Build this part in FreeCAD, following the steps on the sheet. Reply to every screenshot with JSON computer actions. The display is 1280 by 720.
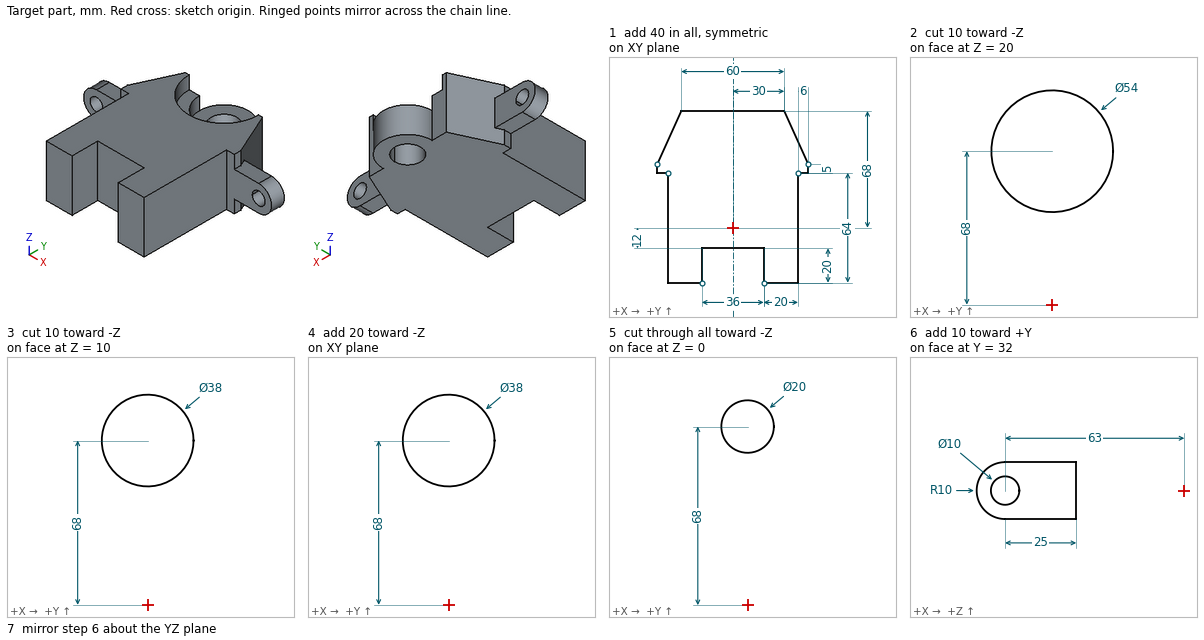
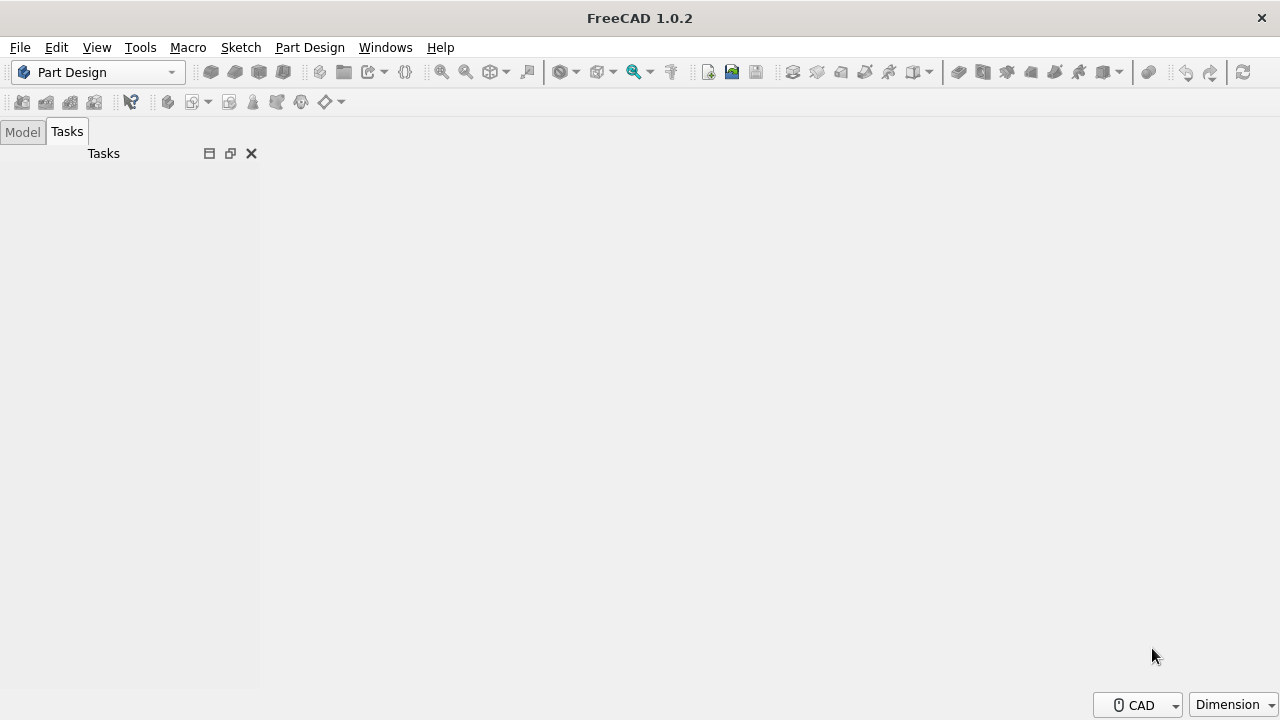
{"action": "left_click", "coordinate": [708, 72]}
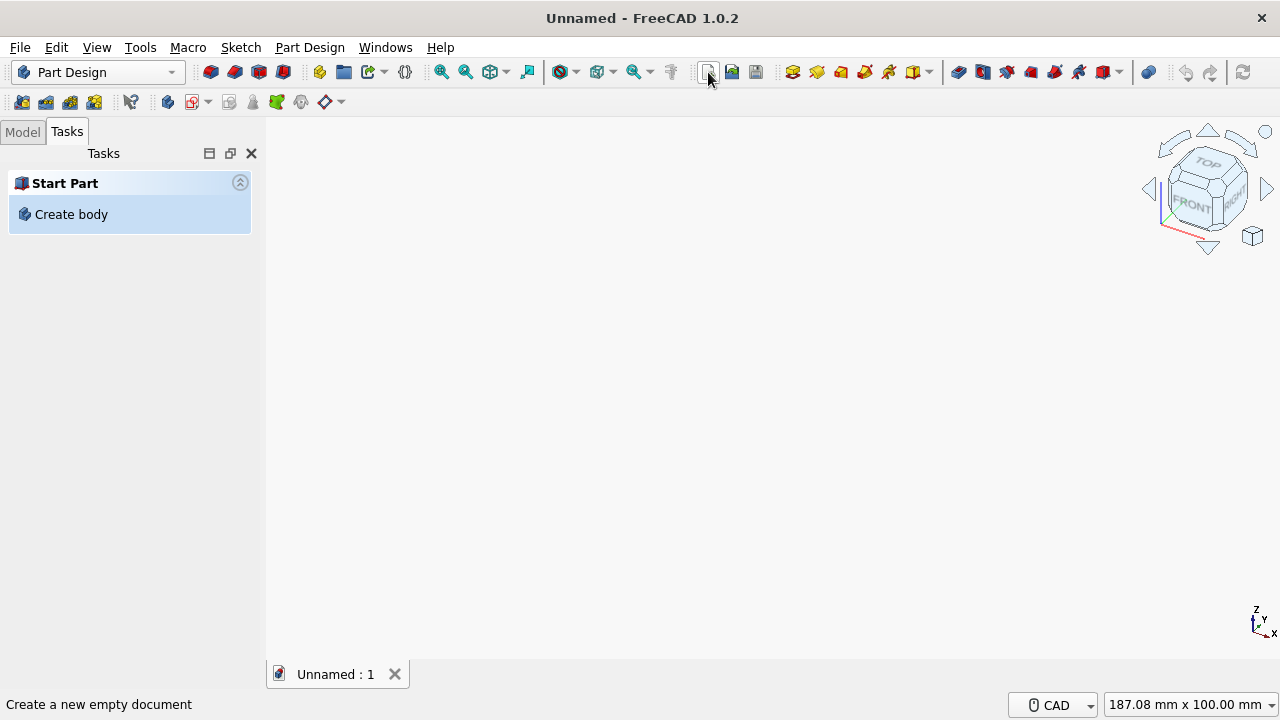
{"action": "left_click", "coordinate": [192, 102]}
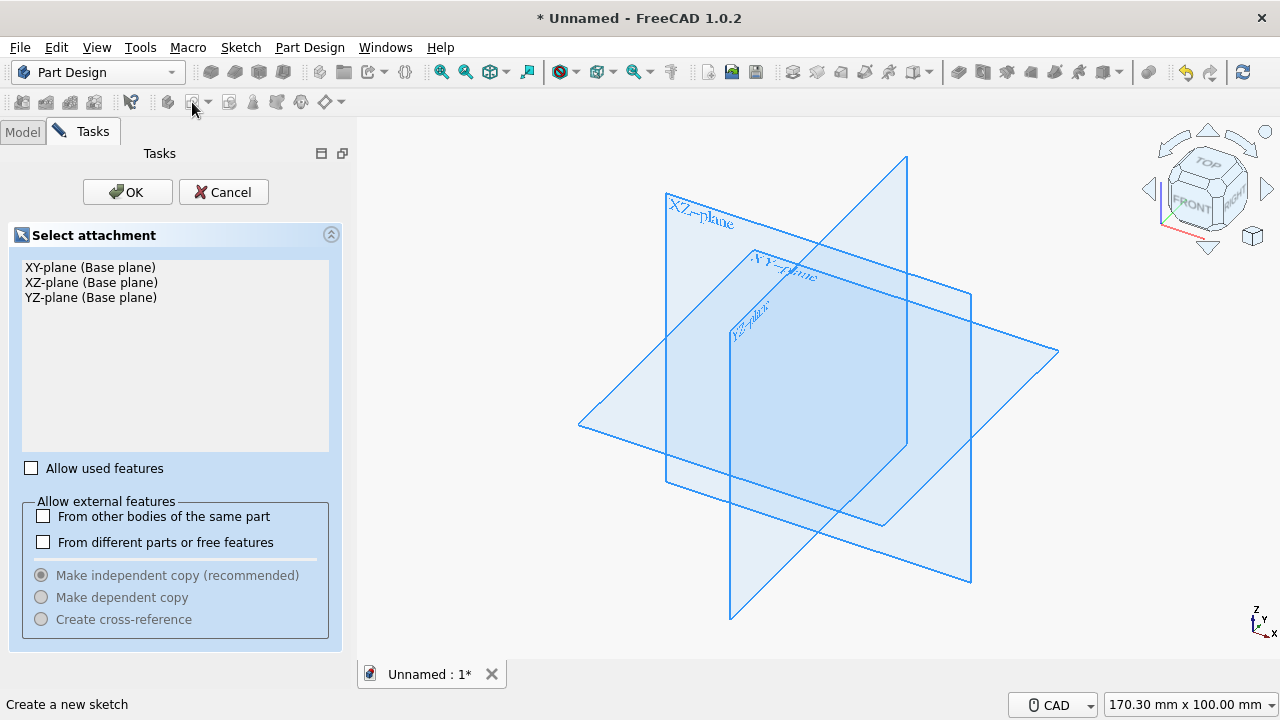
{"action": "left_click", "coordinate": [82, 268]}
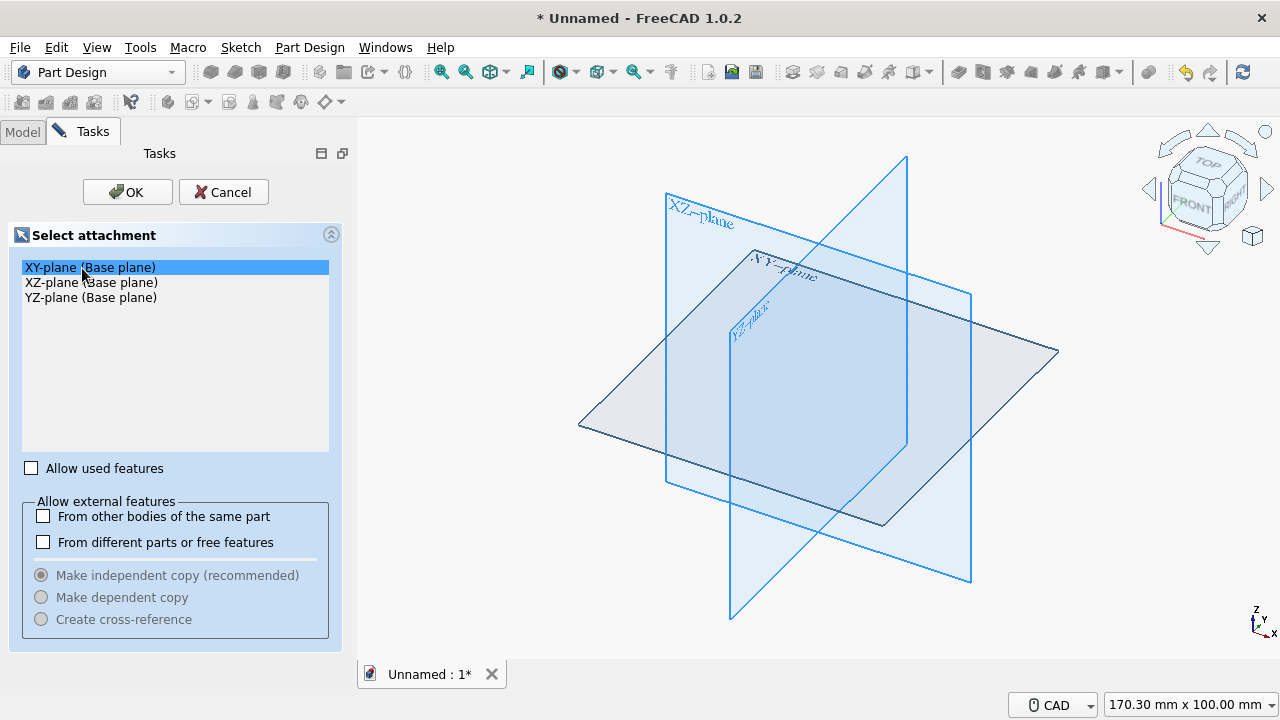
{"action": "left_click", "coordinate": [128, 192]}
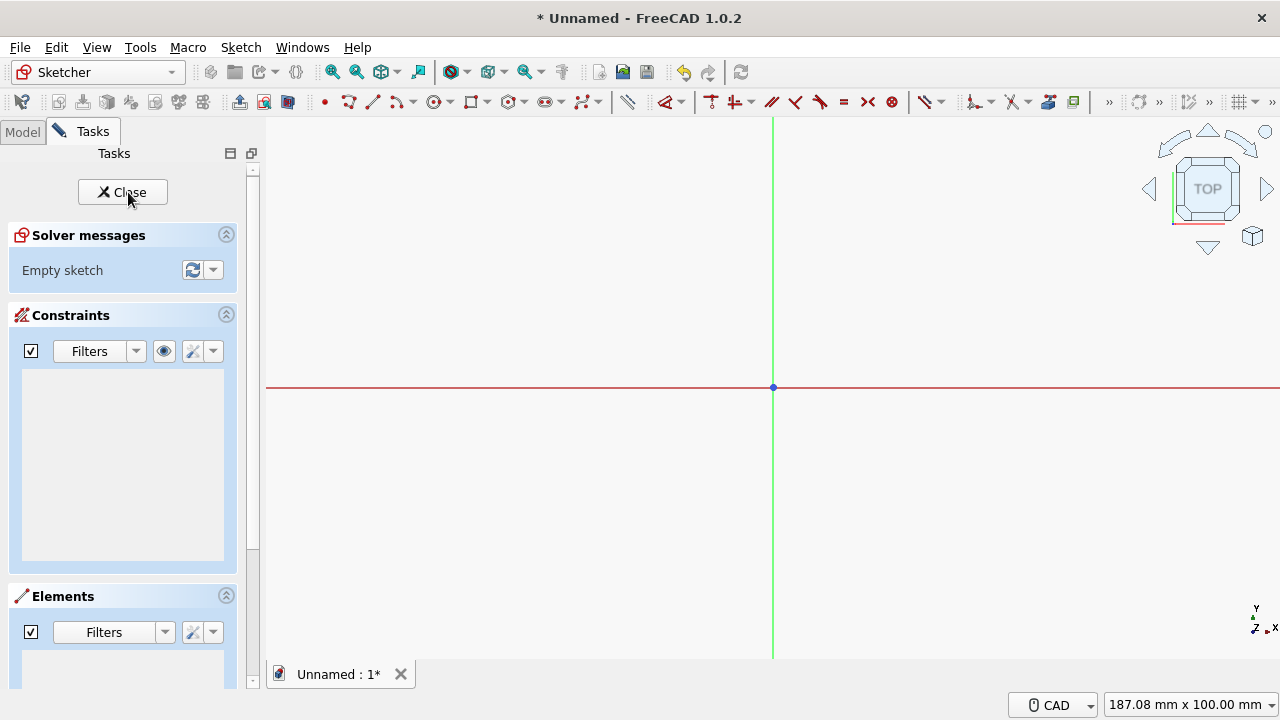
{"action": "scroll", "coordinate": [565, 586], "scroll_direction": "down", "scroll_amount": 2}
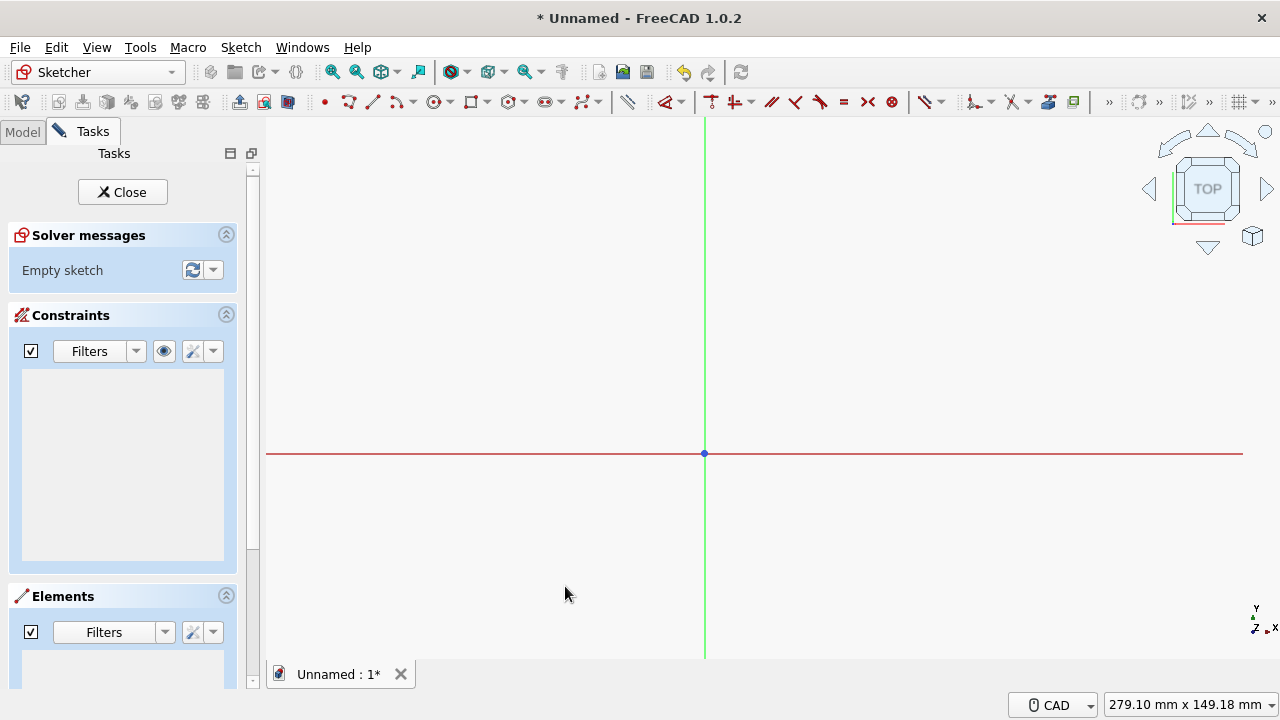
{"action": "left_click", "coordinate": [350, 102]}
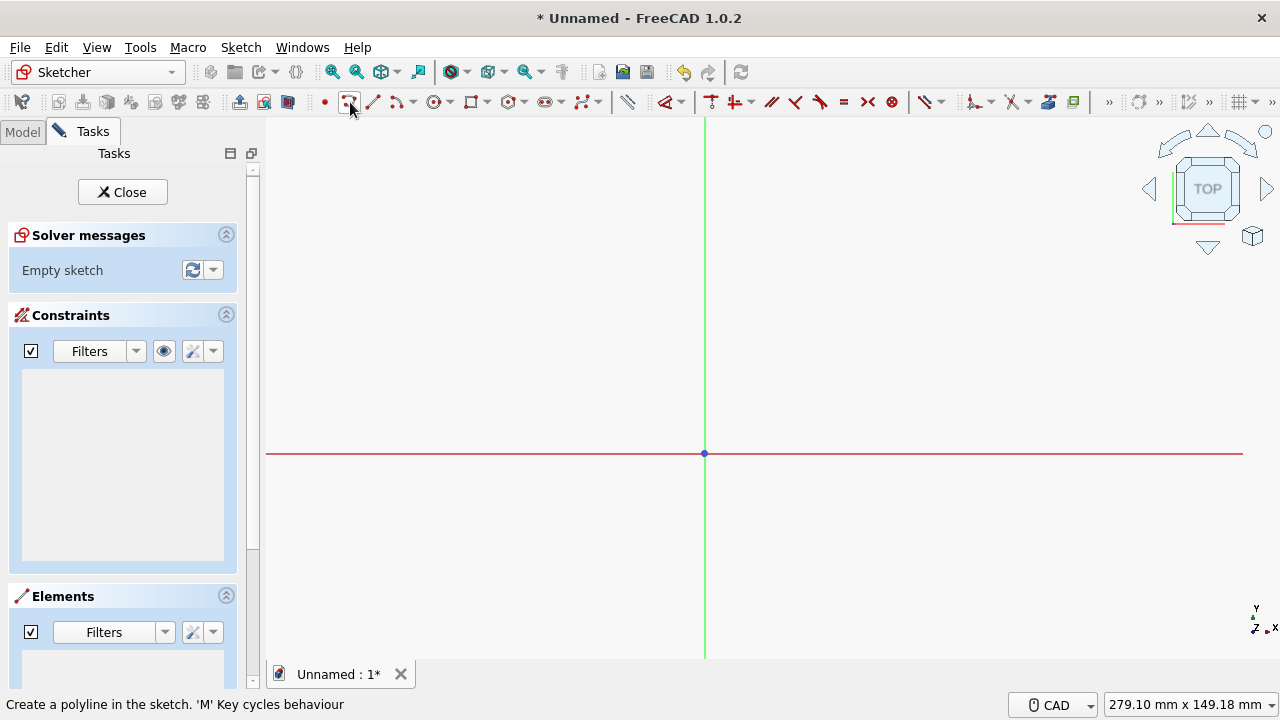
{"action": "left_click", "coordinate": [639, 497]}
{"action": "left_click", "coordinate": [770, 497]}
{"action": "left_click", "coordinate": [770, 570]}
{"action": "left_click", "coordinate": [843, 570]}
{"action": "left_click", "coordinate": [843, 337]}
{"action": "left_click", "coordinate": [864, 337]}
{"action": "left_click", "coordinate": [864, 319]}
{"action": "left_click", "coordinate": [814, 207]}
{"action": "left_click", "coordinate": [596, 207]}
{"action": "left_click", "coordinate": [545, 319]}
{"action": "left_click", "coordinate": [545, 337]}
{"action": "left_click", "coordinate": [566, 337]}
{"action": "left_click", "coordinate": [566, 570]}
{"action": "left_click", "coordinate": [639, 570]}
{"action": "left_click", "coordinate": [639, 498]}
{"action": "key", "text": "Escape"}
{"action": "key", "text": "Escape"}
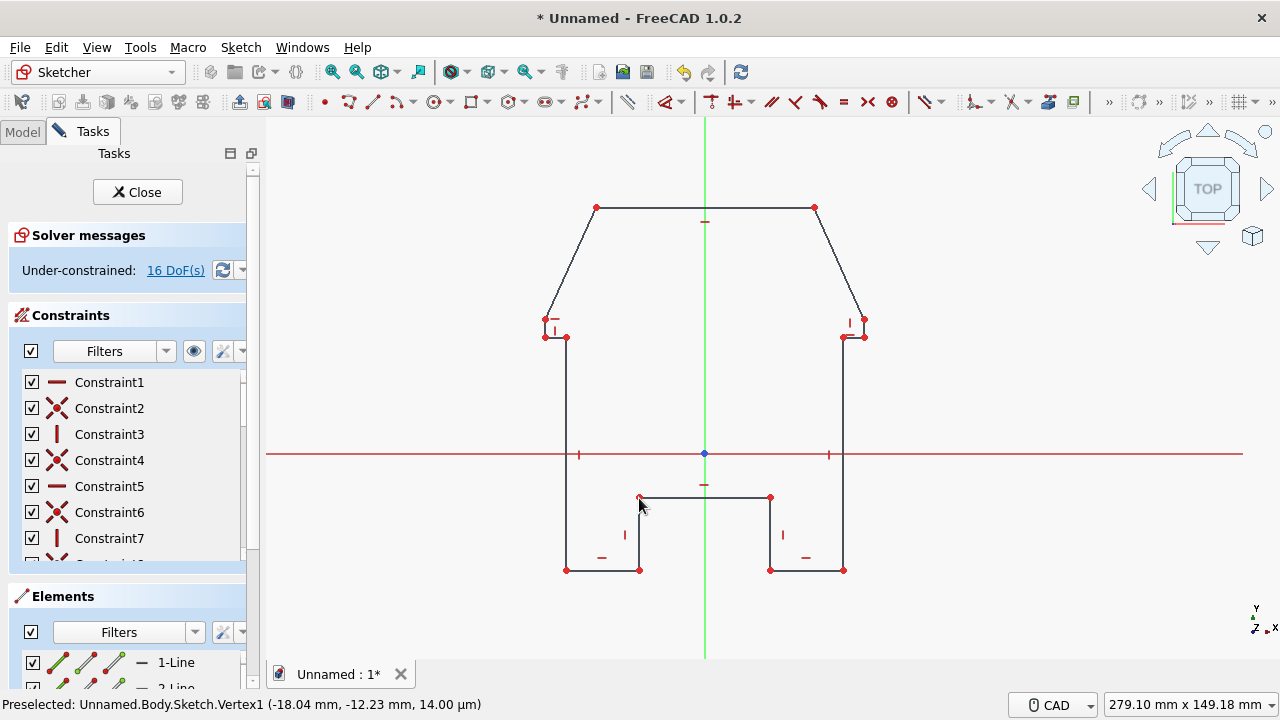
{"action": "left_click", "coordinate": [864, 320]}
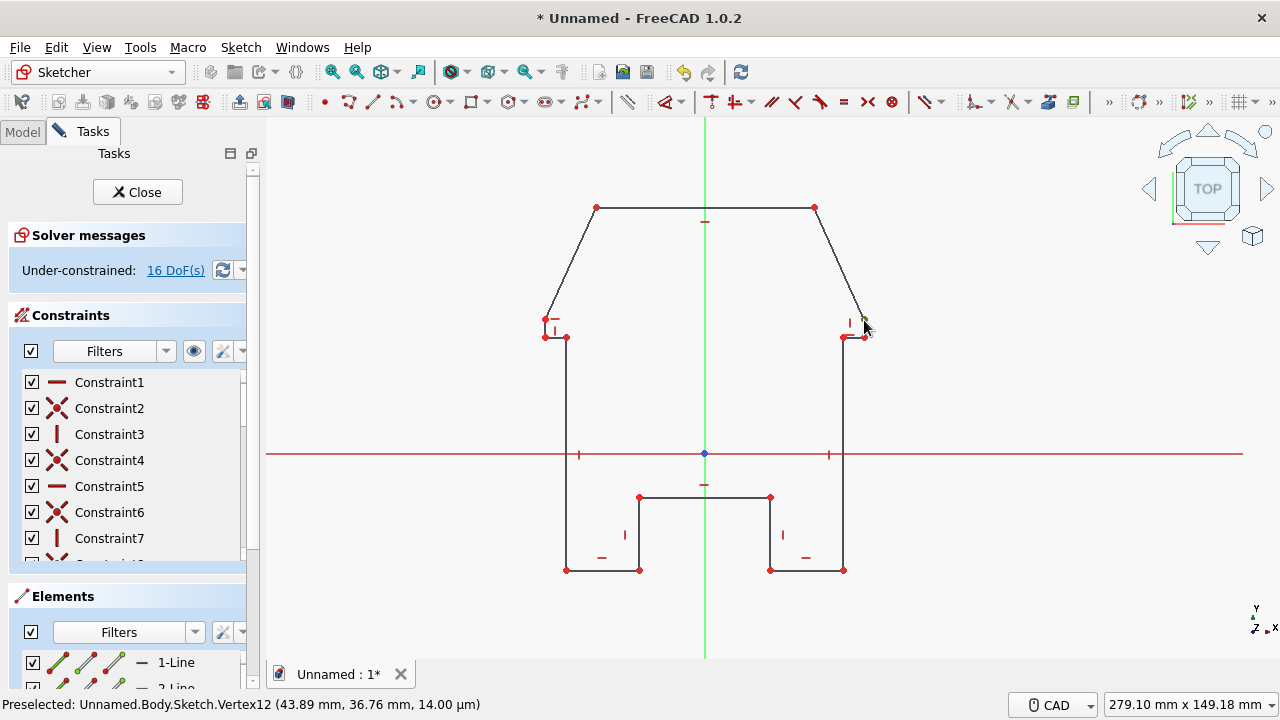
{"action": "left_click", "coordinate": [545, 320]}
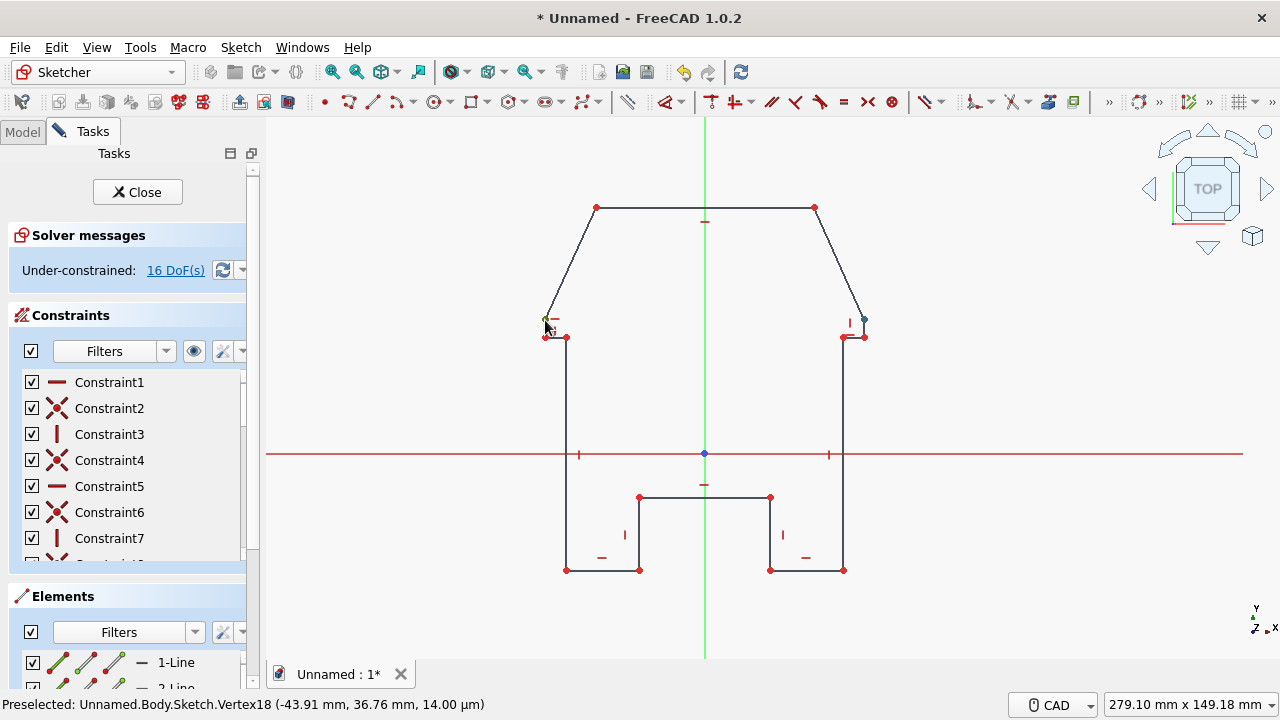
{"action": "left_click", "coordinate": [705, 596]}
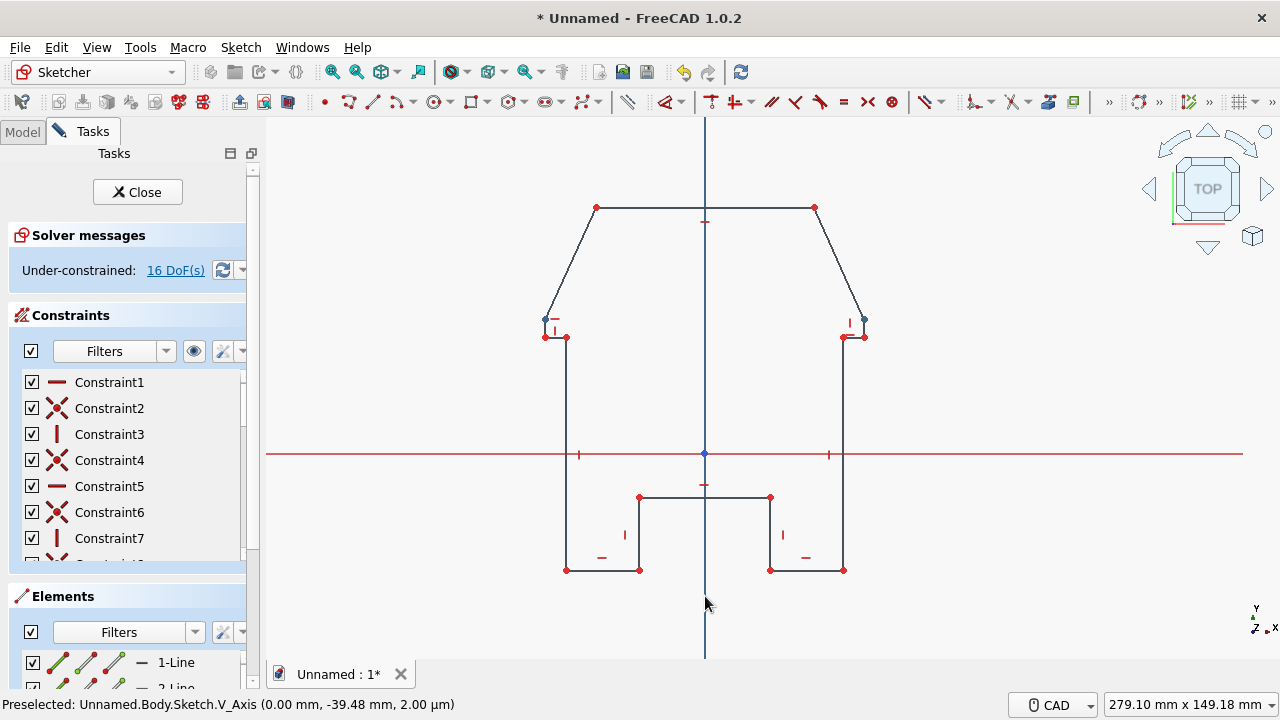
{"action": "left_click", "coordinate": [868, 102]}